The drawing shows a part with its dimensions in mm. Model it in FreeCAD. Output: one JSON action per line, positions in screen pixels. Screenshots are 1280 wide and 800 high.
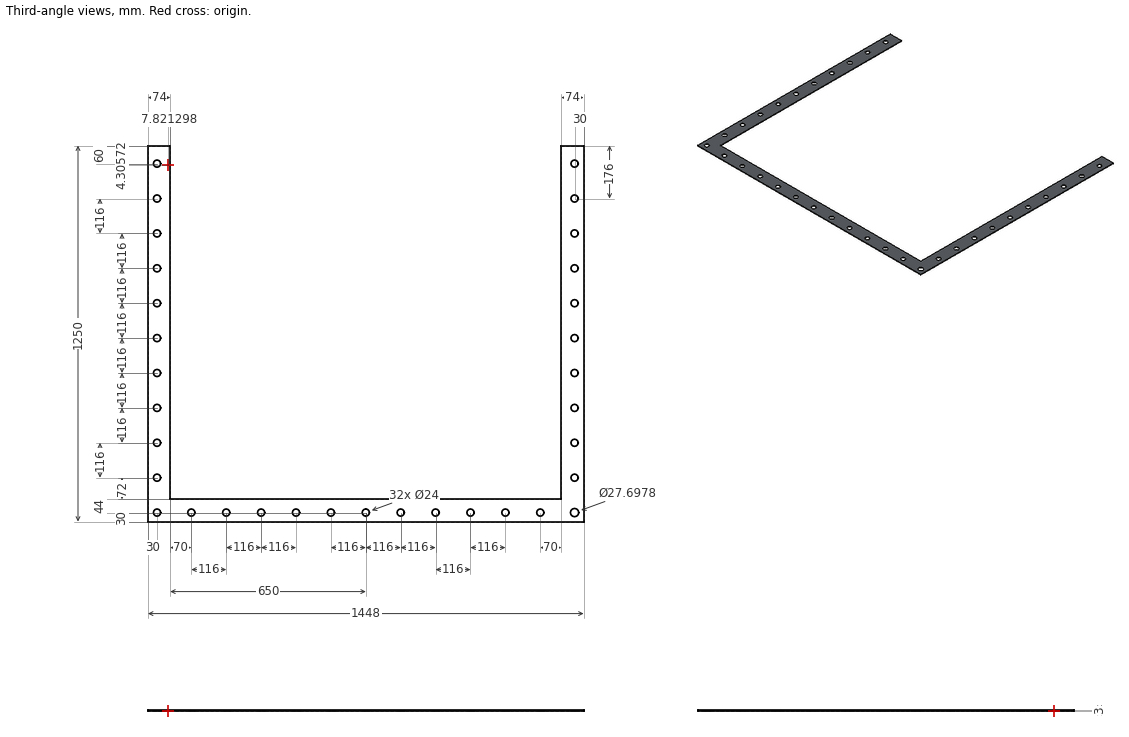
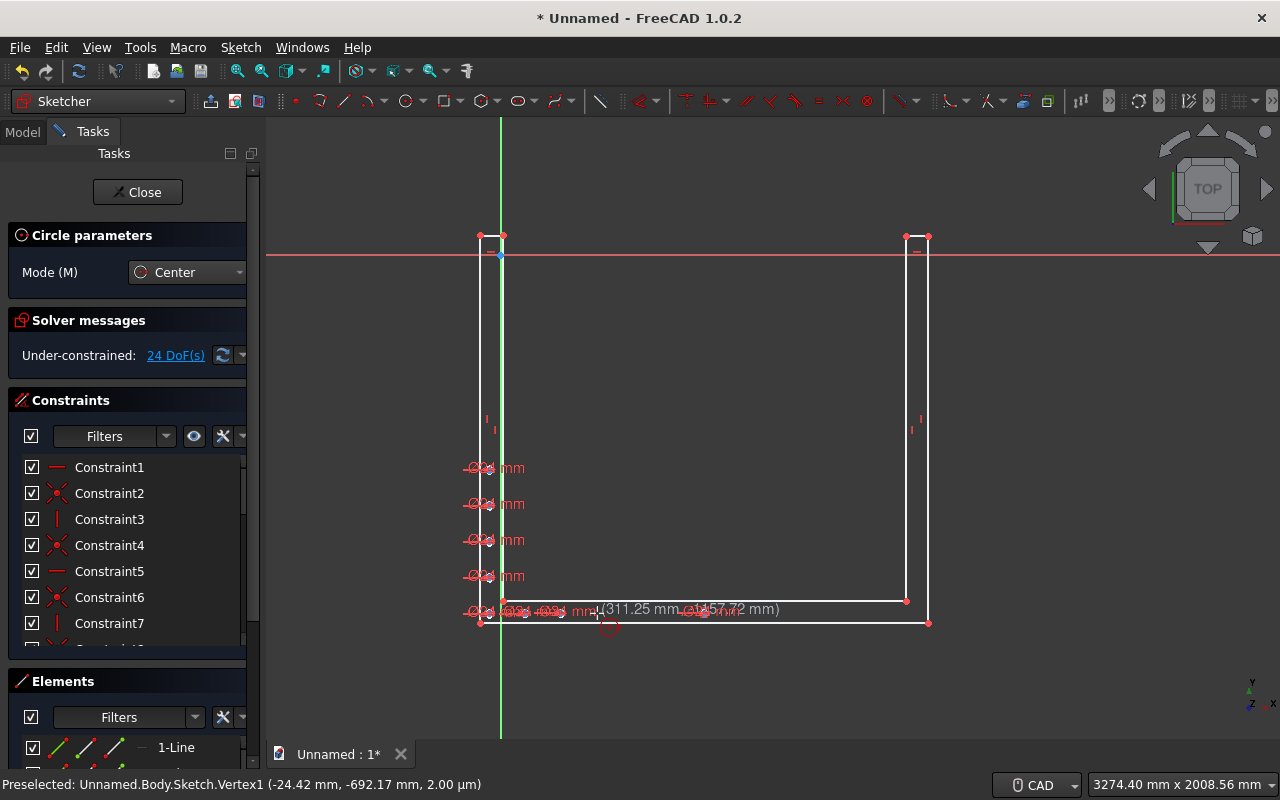
{"action": "scroll", "coordinate": [597, 613], "scroll_direction": "up", "scroll_amount": 3}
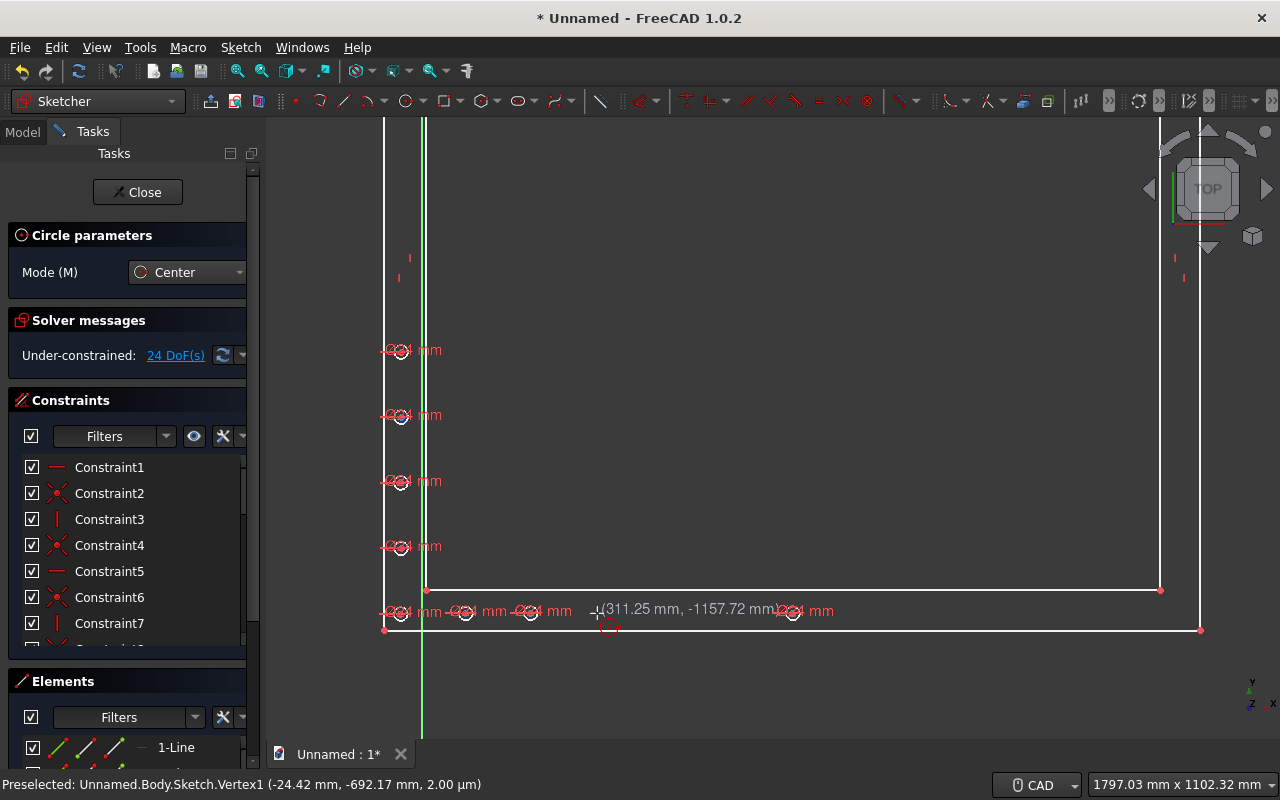
{"action": "left_click", "coordinate": [596, 613]}
{"action": "mouse_move", "coordinate": [601, 608]}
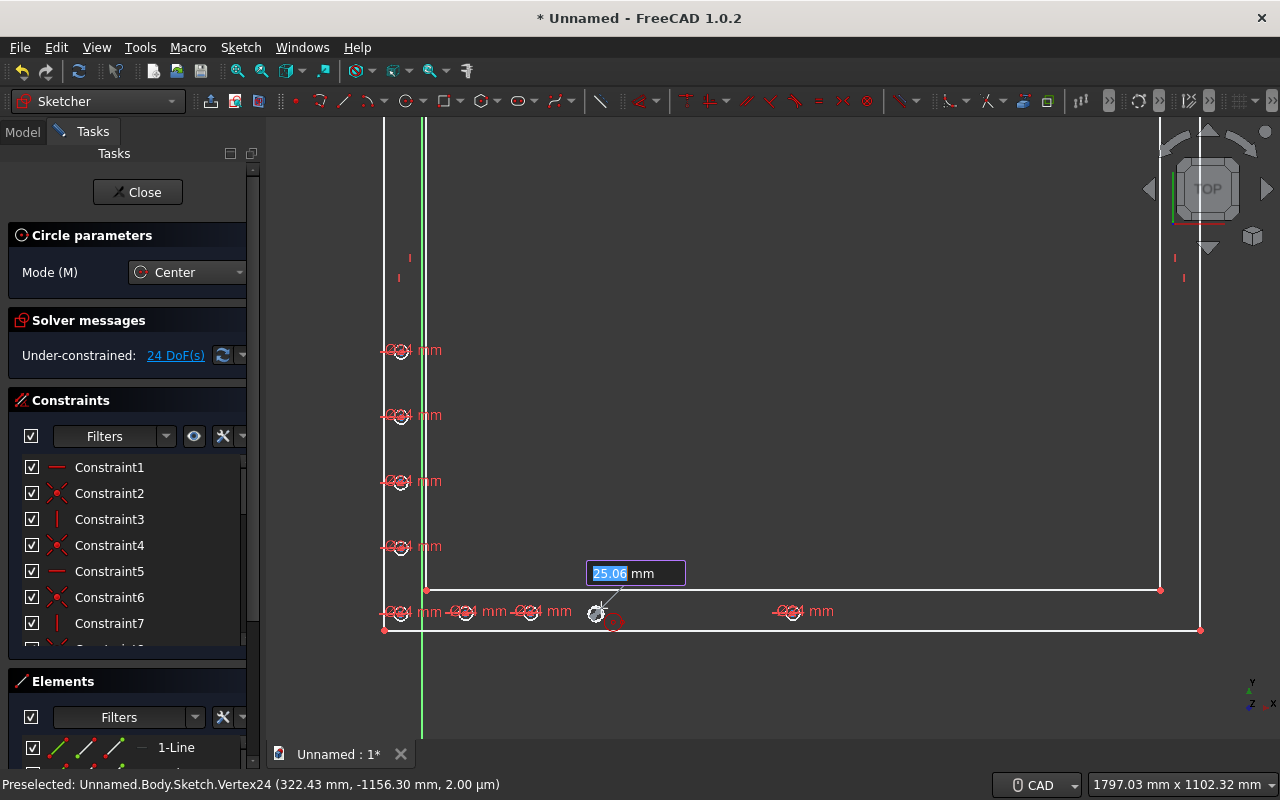
{"action": "type", "text": "24"}
{"action": "key", "text": "Return"}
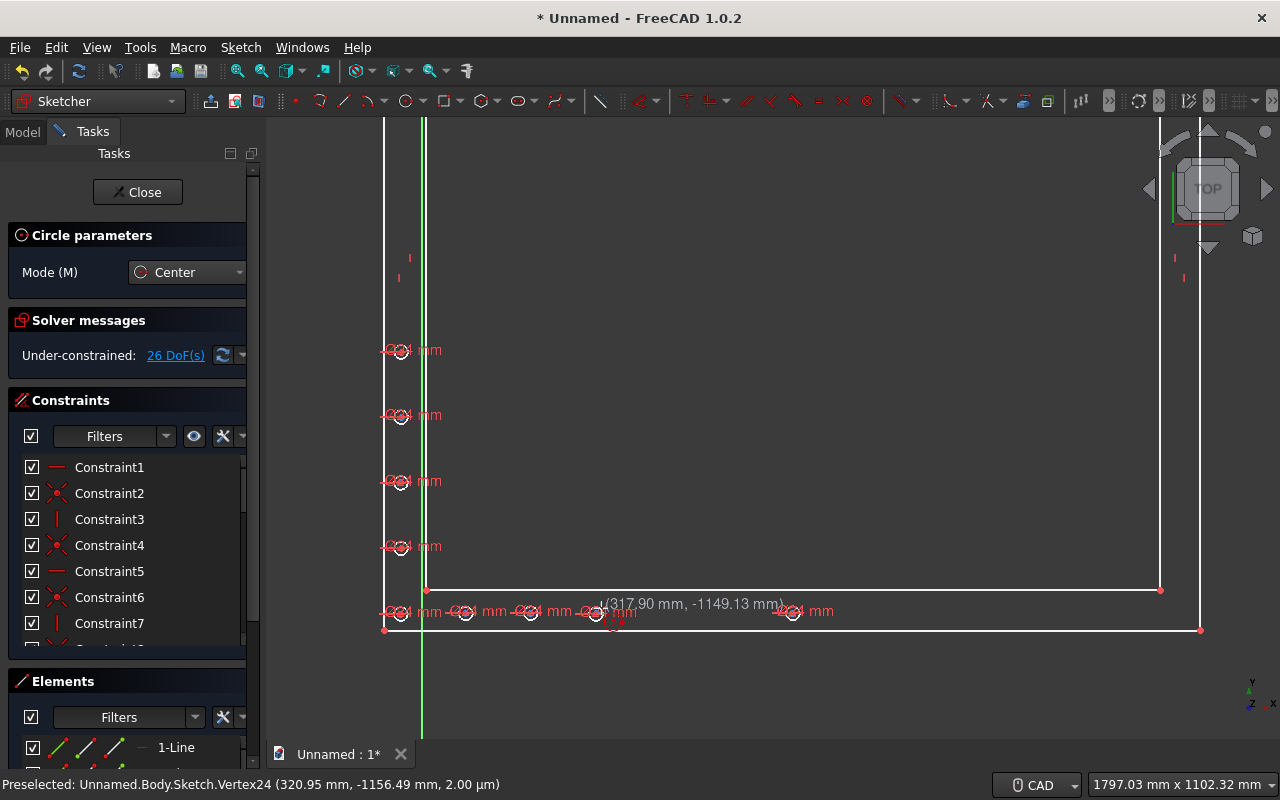
{"action": "scroll", "coordinate": [662, 613], "scroll_direction": "up", "scroll_amount": 7}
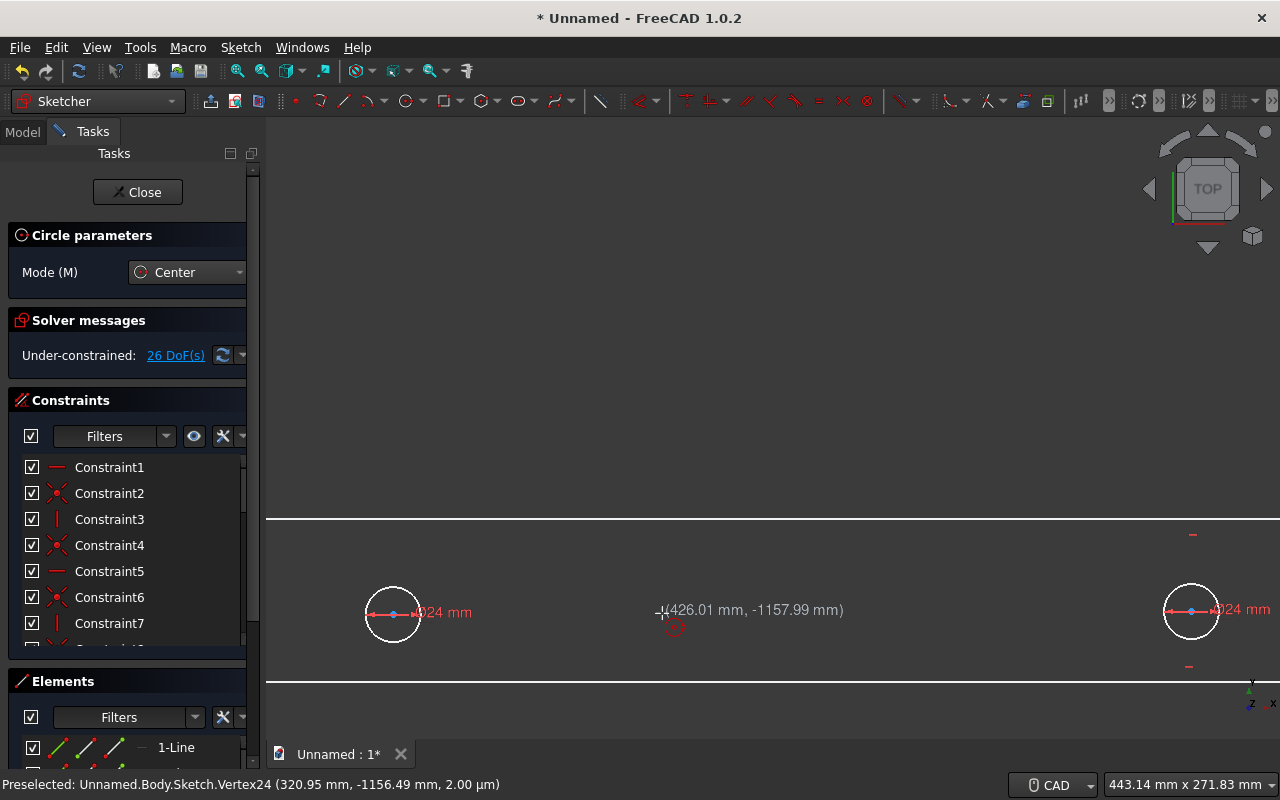
{"action": "scroll", "coordinate": [628, 613], "scroll_direction": "down", "scroll_amount": 10}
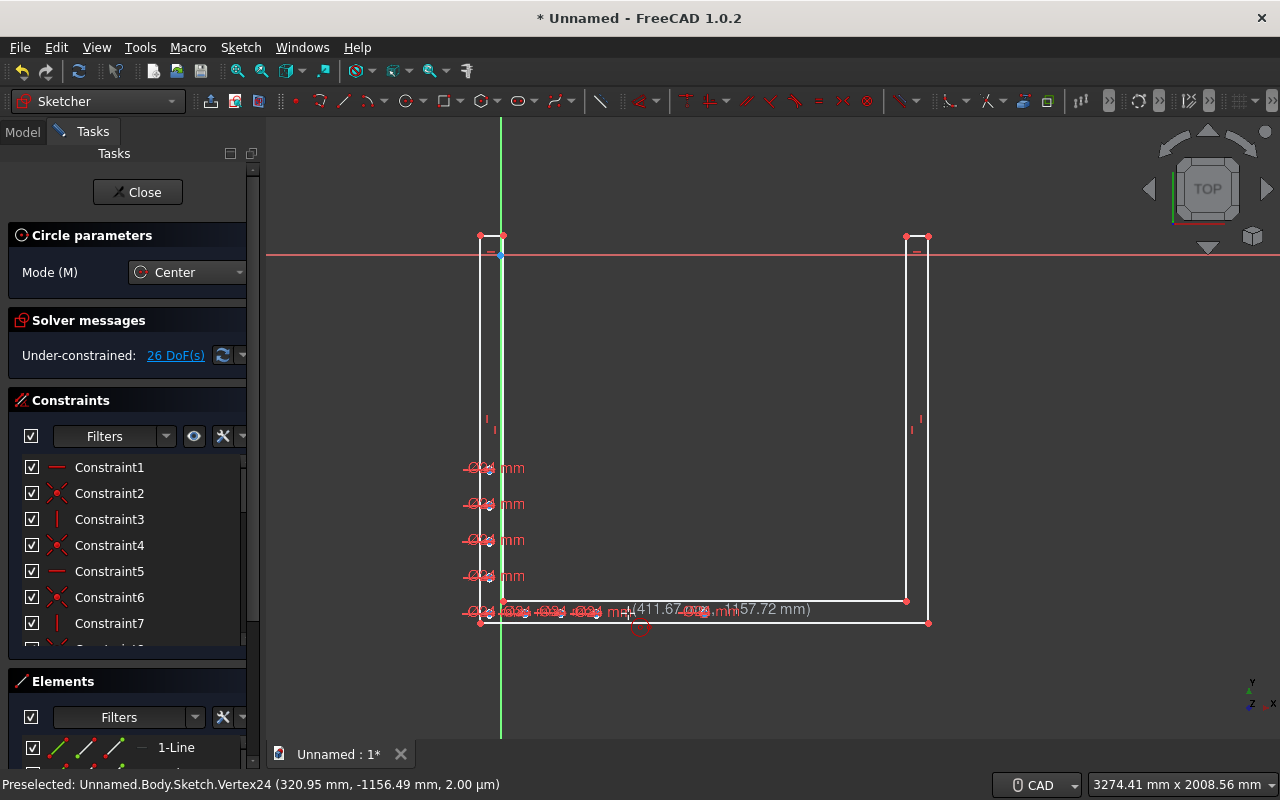
{"action": "scroll", "coordinate": [633, 613], "scroll_direction": "up", "scroll_amount": 3}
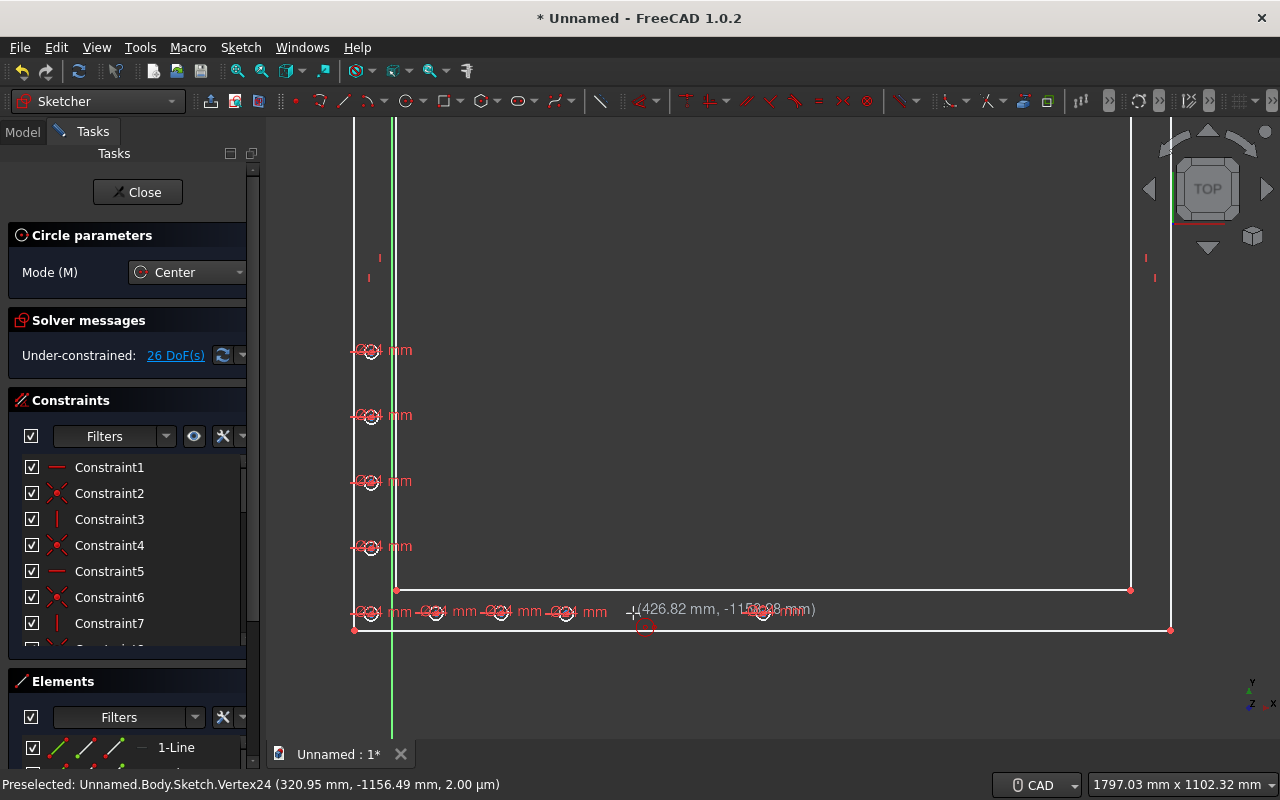
{"action": "left_click", "coordinate": [632, 613]}
{"action": "mouse_move", "coordinate": [637, 608]}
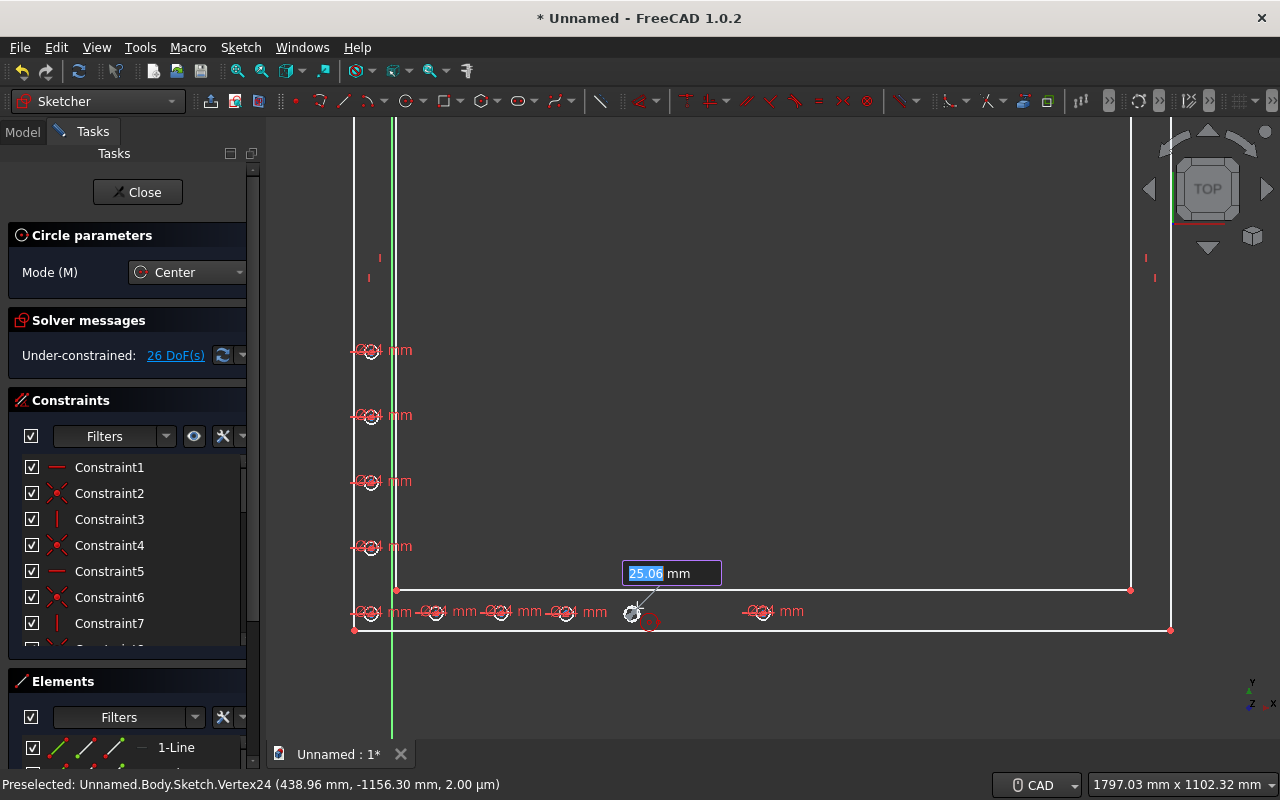
{"action": "type", "text": "24"}
{"action": "key", "text": "Return"}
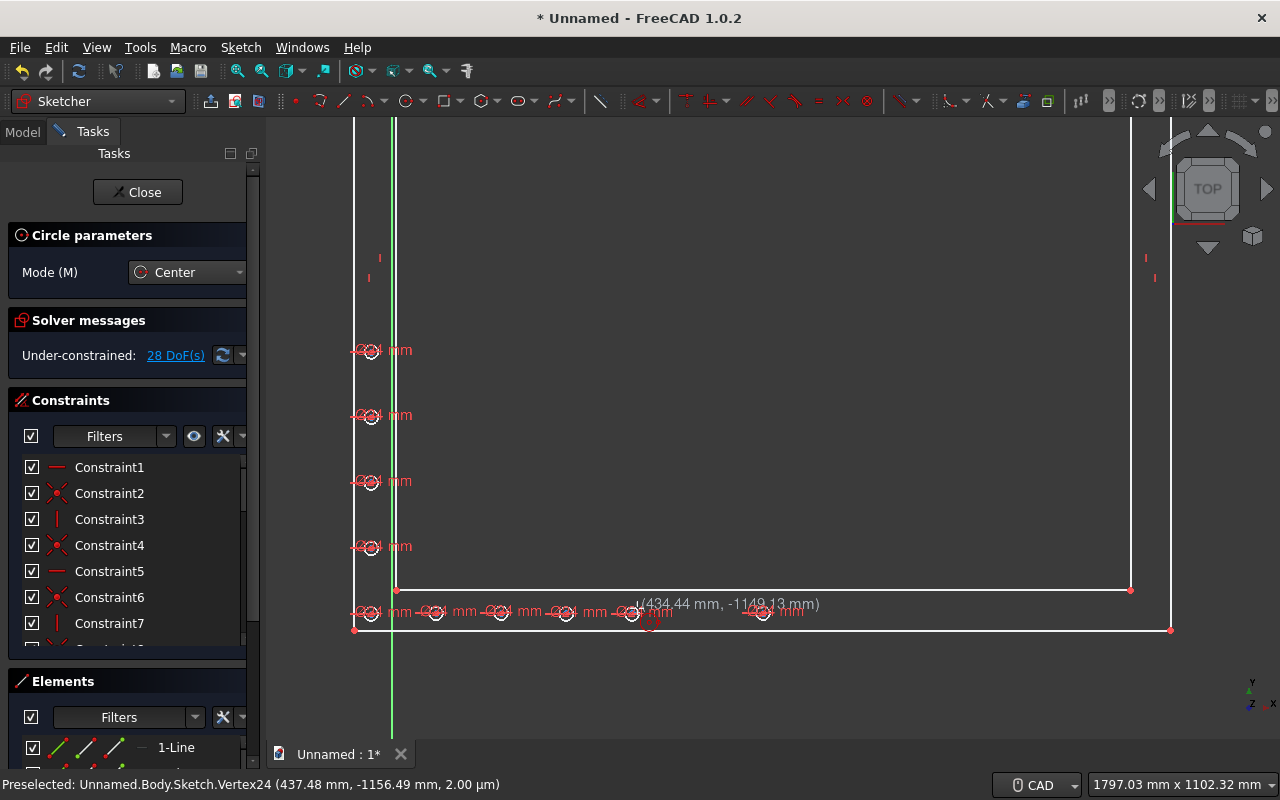
{"action": "scroll", "coordinate": [698, 613], "scroll_direction": "up", "scroll_amount": 7}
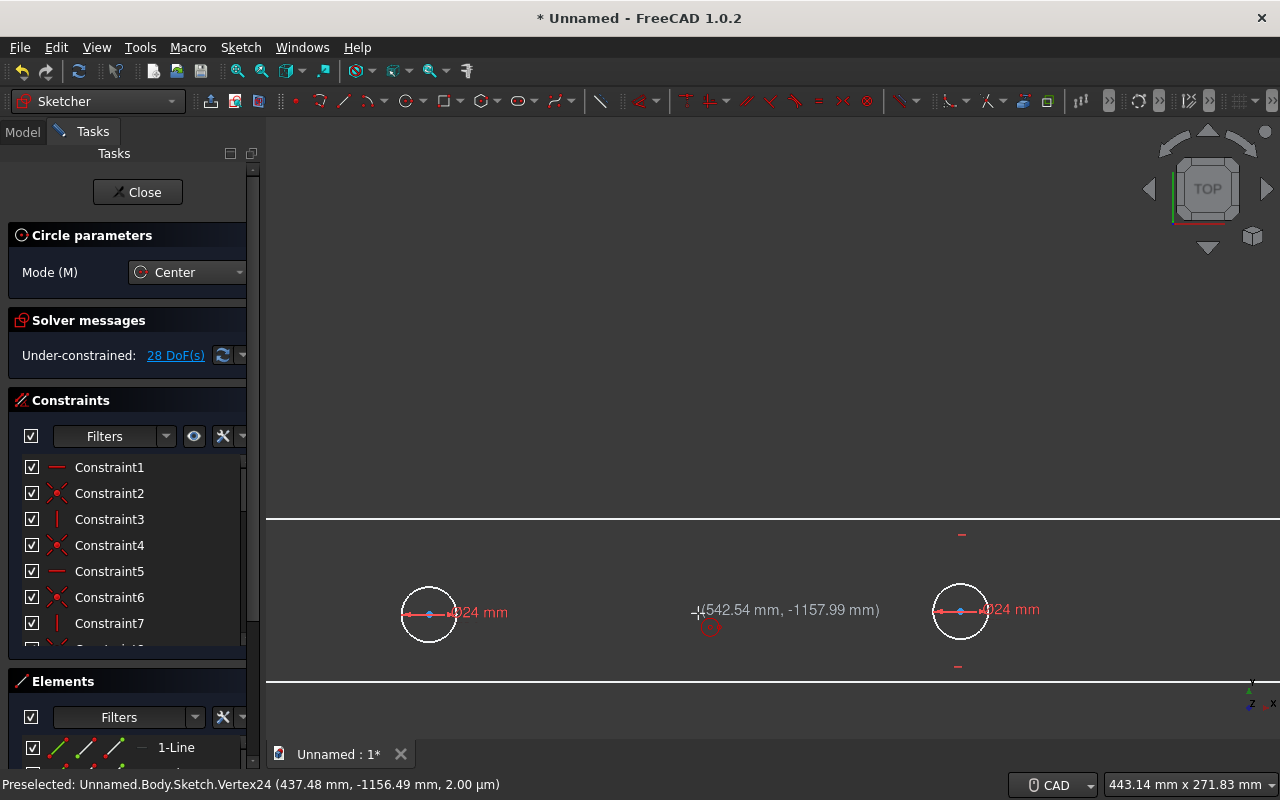
{"action": "scroll", "coordinate": [664, 613], "scroll_direction": "down", "scroll_amount": 10}